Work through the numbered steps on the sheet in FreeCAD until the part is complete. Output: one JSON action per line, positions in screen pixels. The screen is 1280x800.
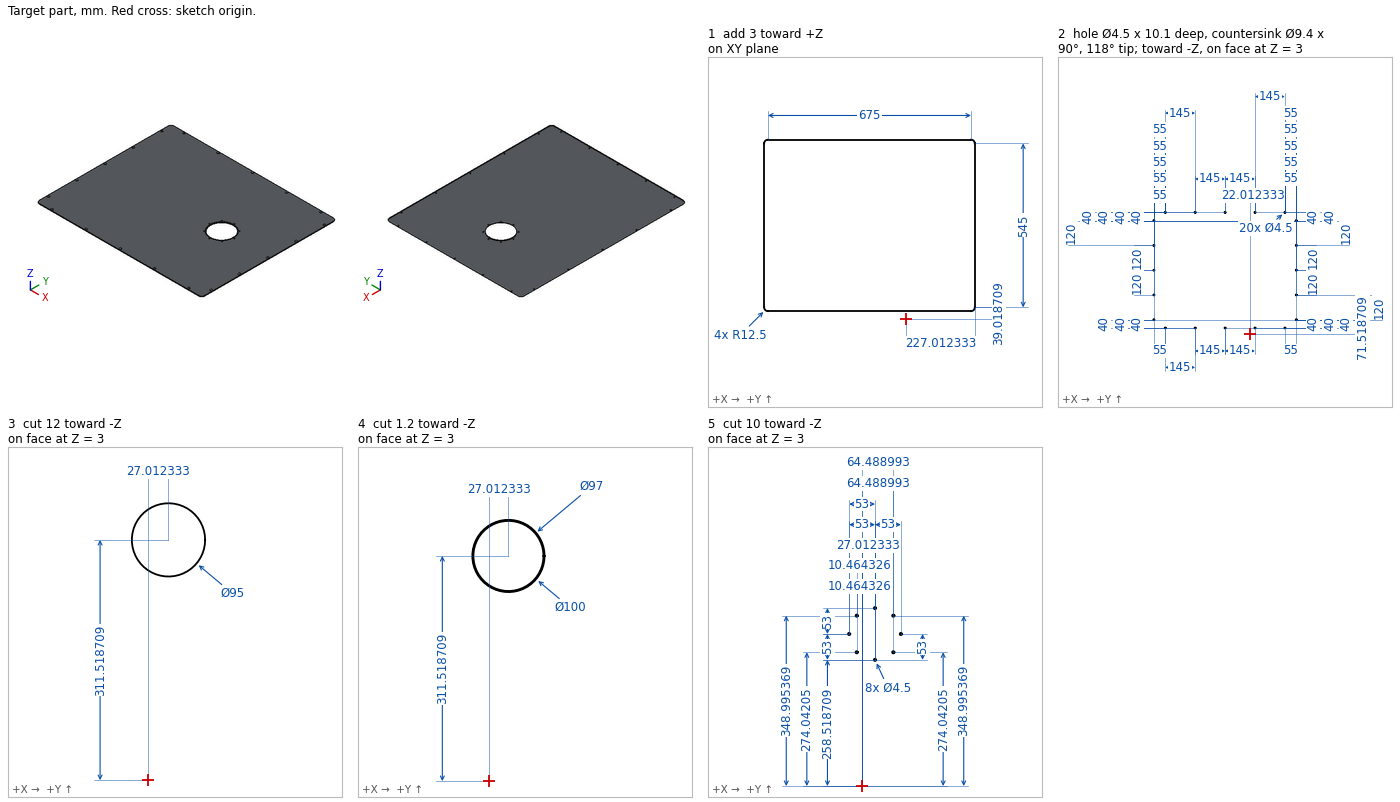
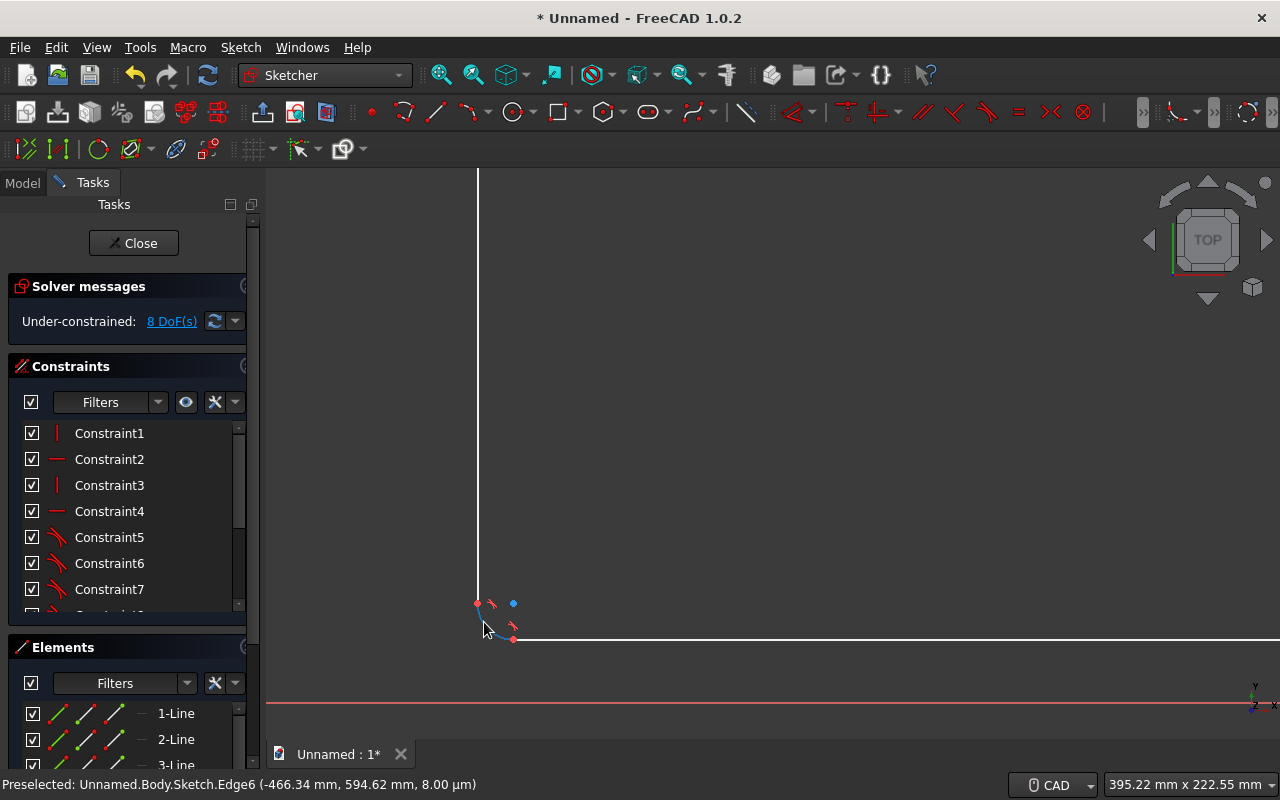
{"action": "left_click", "coordinate": [482, 620]}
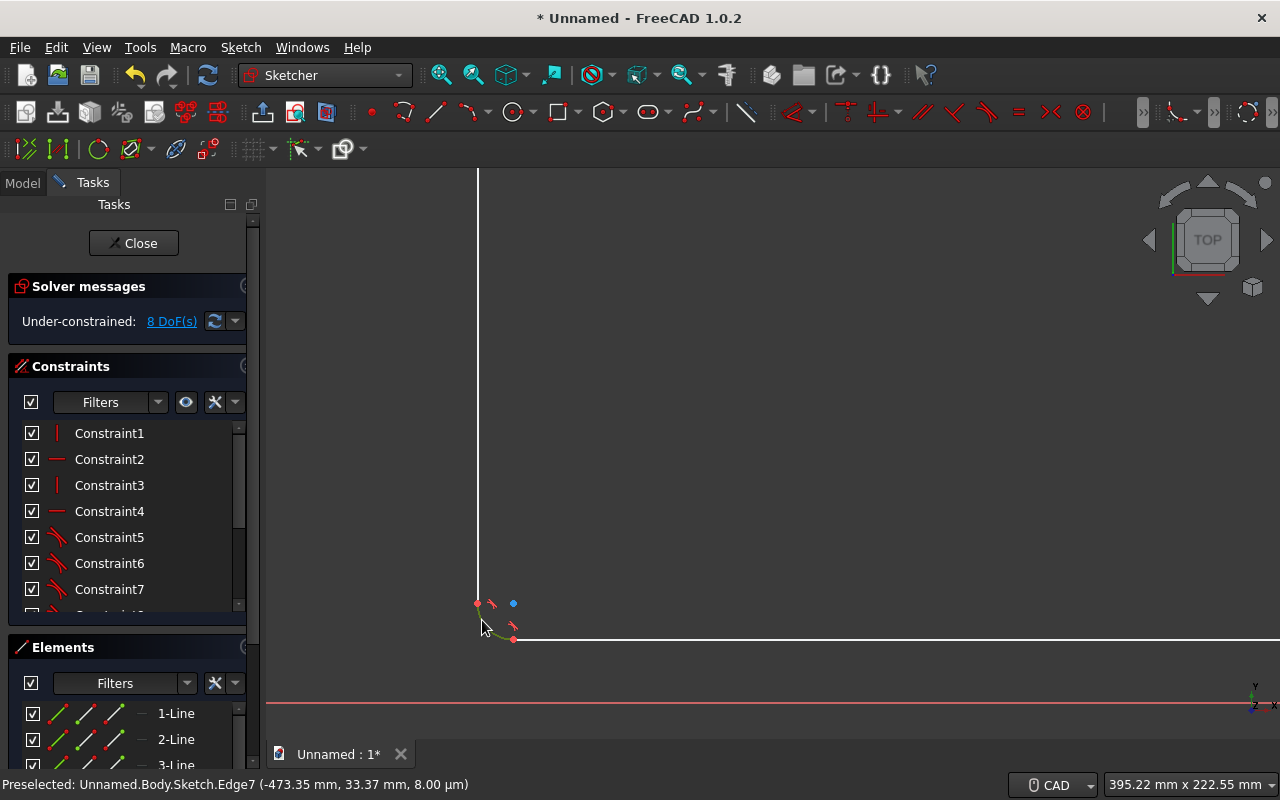
{"action": "scroll", "coordinate": [484, 622], "scroll_direction": "down", "scroll_amount": 7}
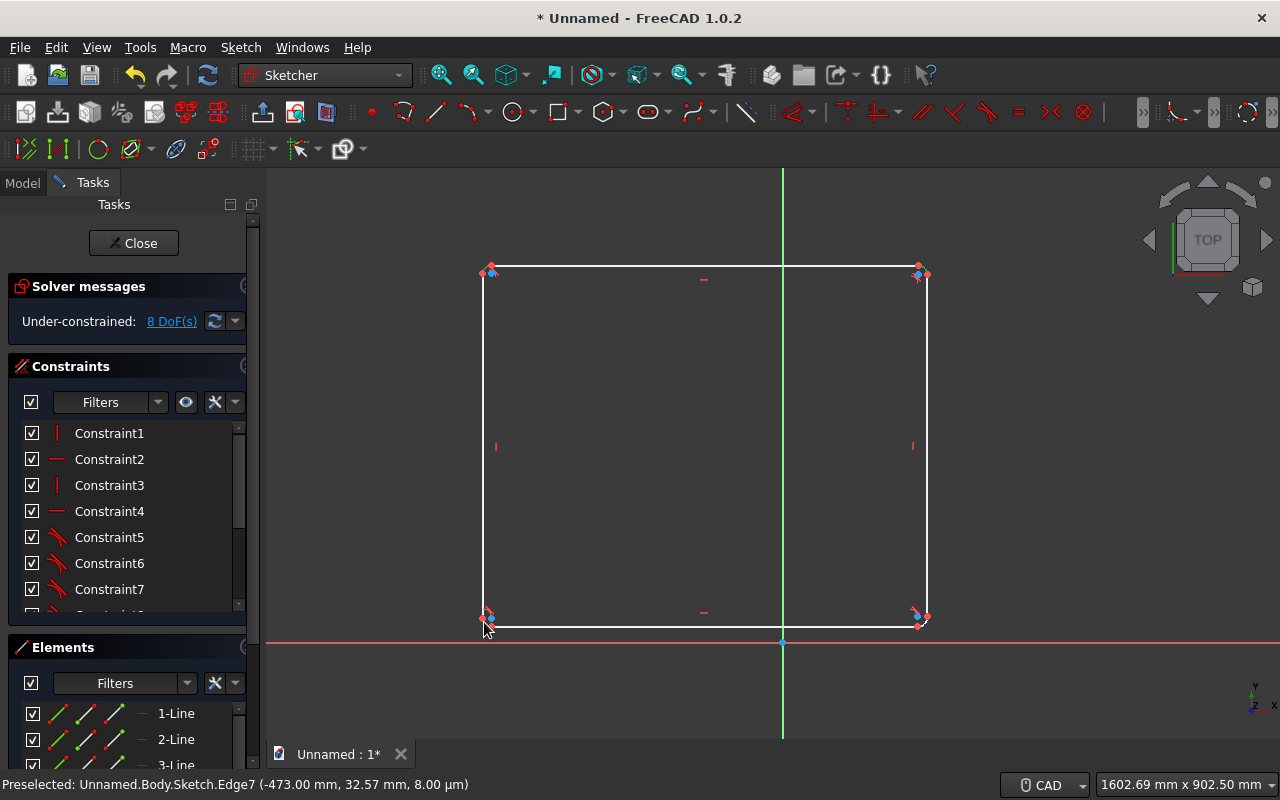
{"action": "scroll", "coordinate": [922, 626], "scroll_direction": "up", "scroll_amount": 6}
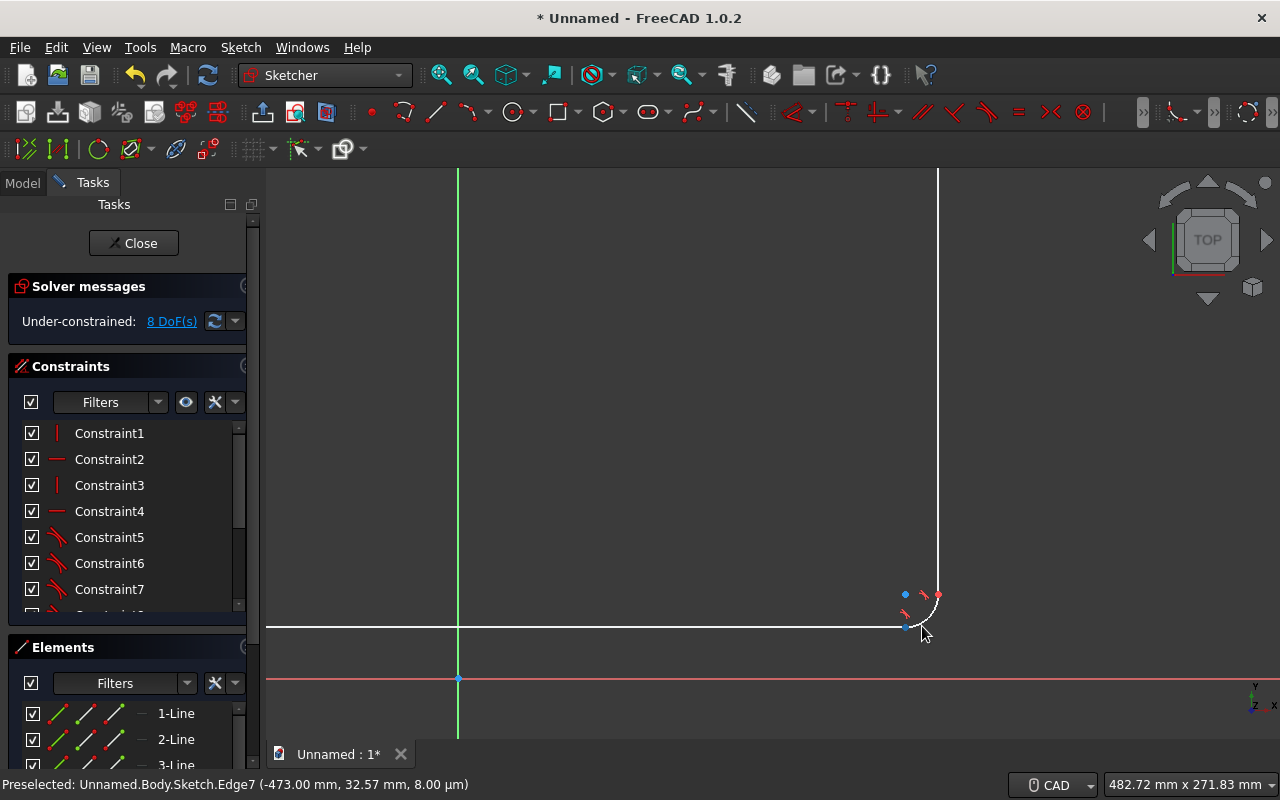
{"action": "left_click", "coordinate": [920, 624]}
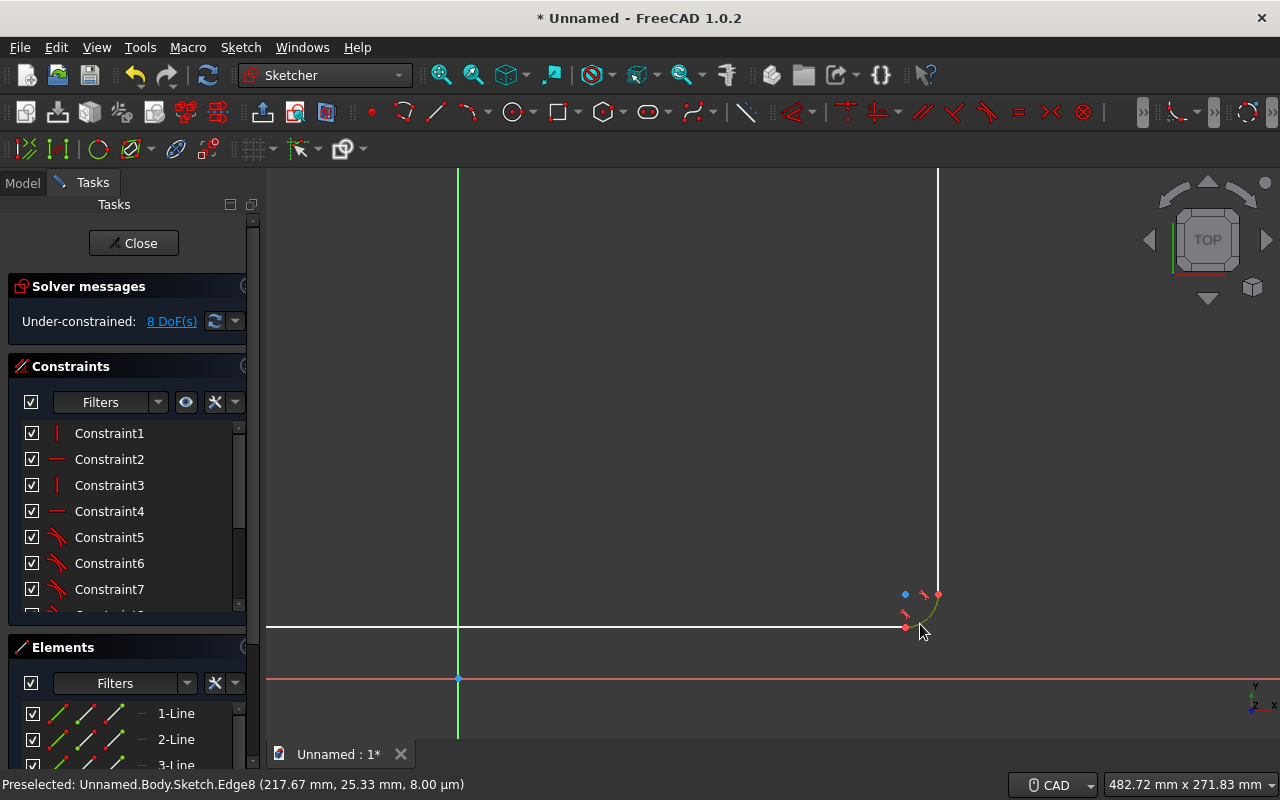
{"action": "left_click", "coordinate": [1020, 112]}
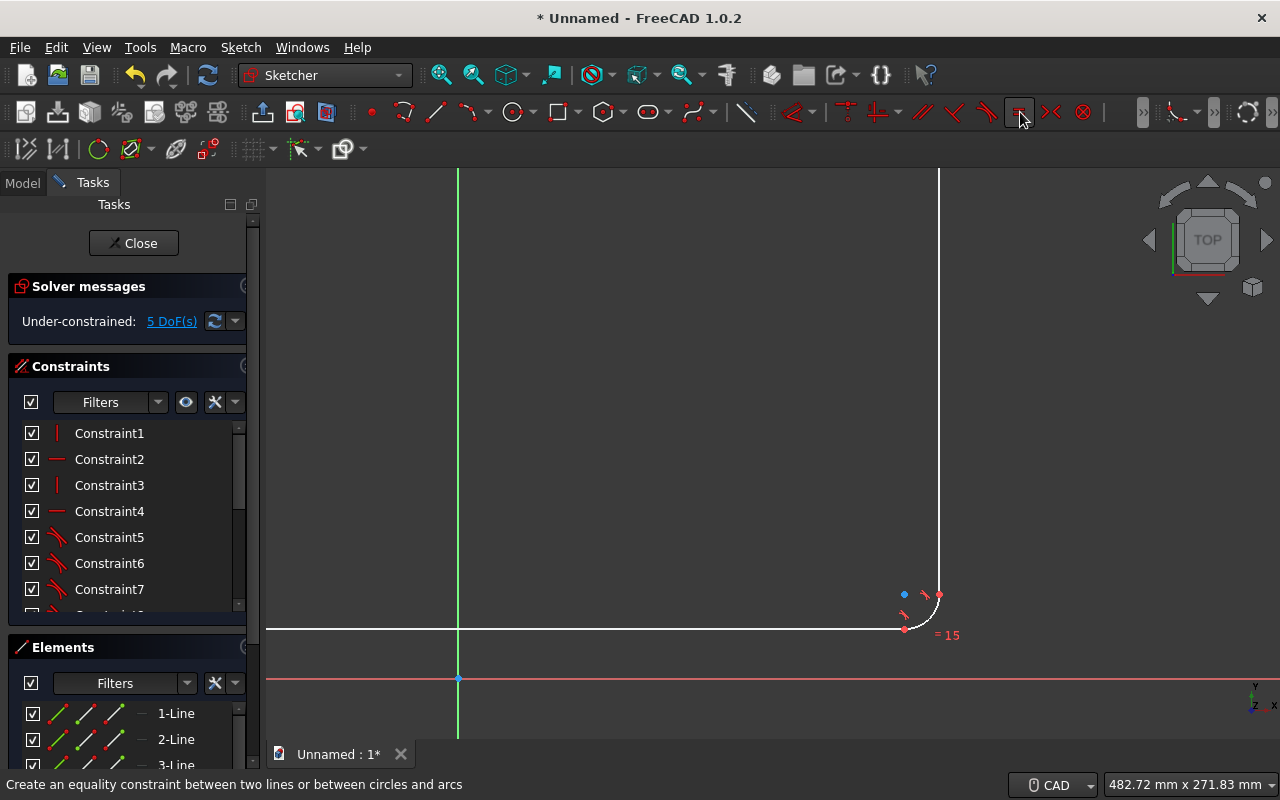
{"action": "scroll", "coordinate": [922, 626], "scroll_direction": "down", "scroll_amount": 6}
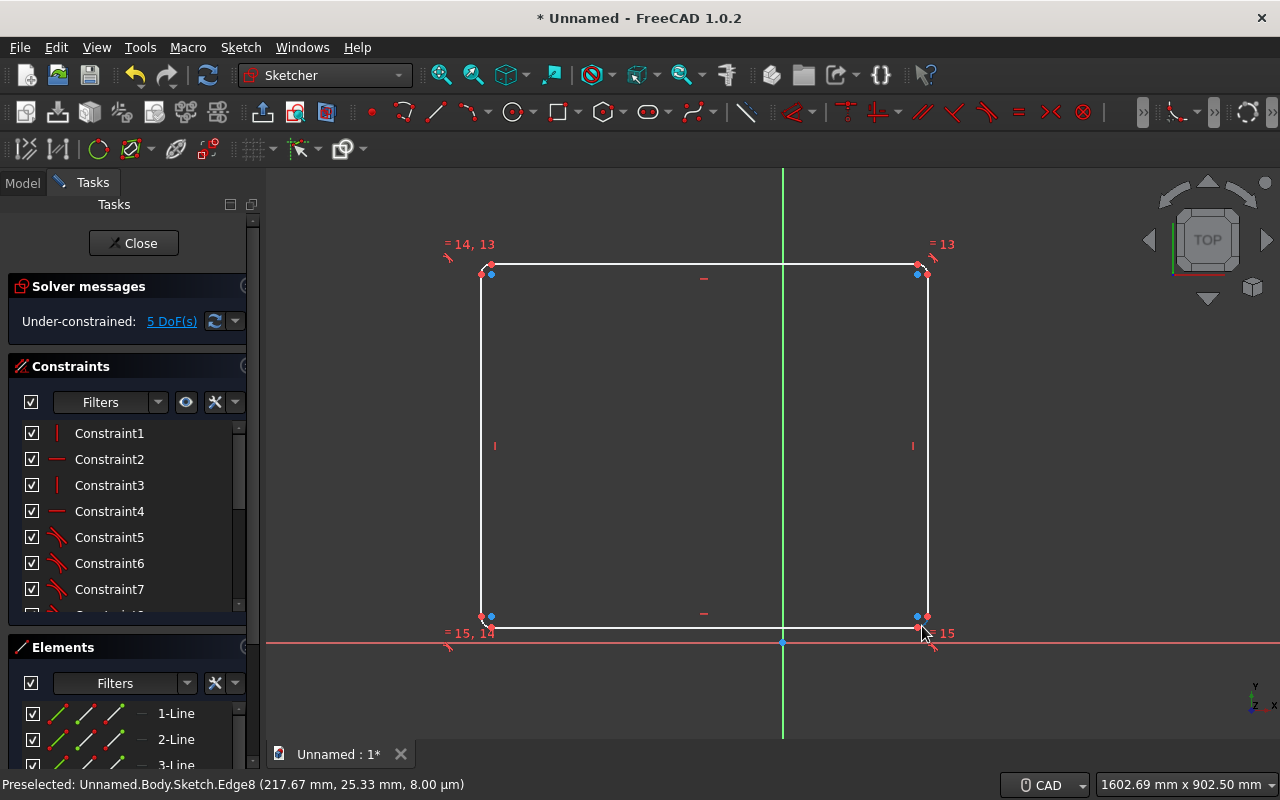
{"action": "scroll", "coordinate": [927, 270], "scroll_direction": "up", "scroll_amount": 9}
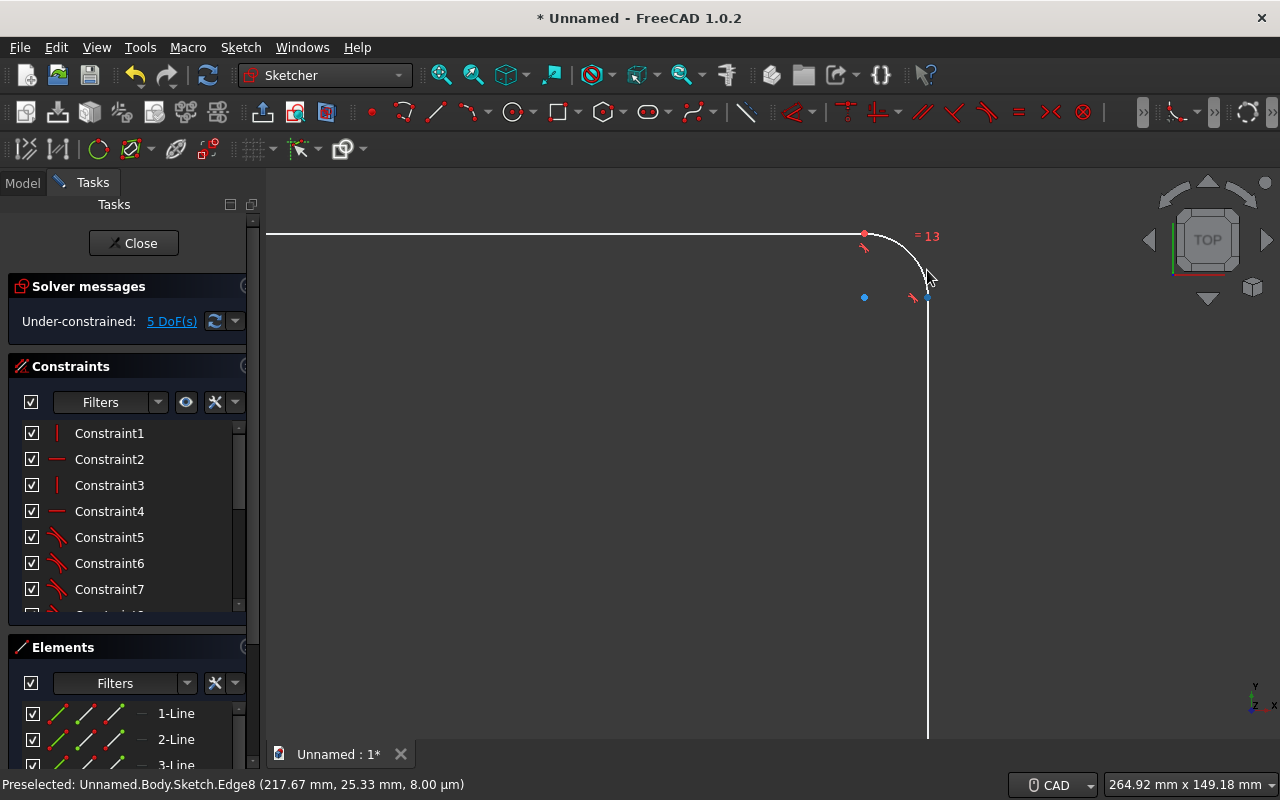
{"action": "left_click", "coordinate": [921, 269]}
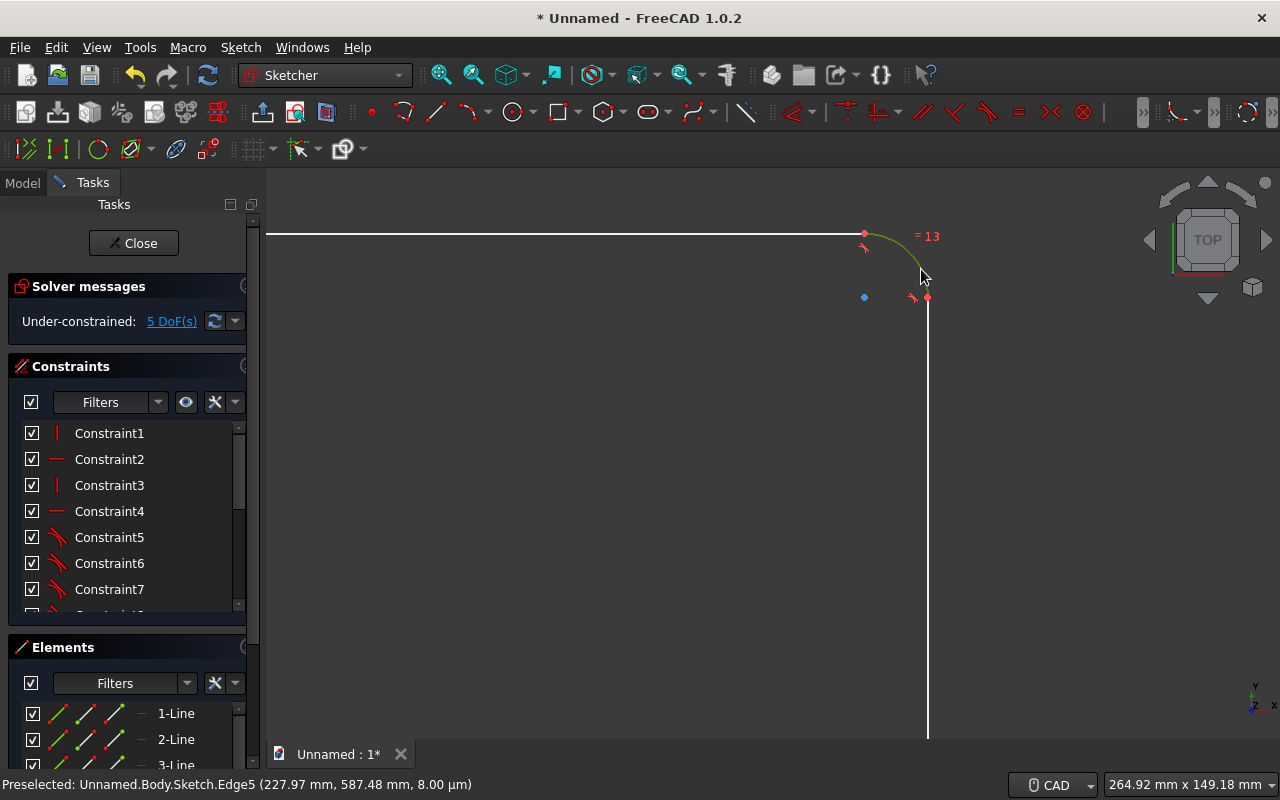
{"action": "left_click", "coordinate": [814, 112]}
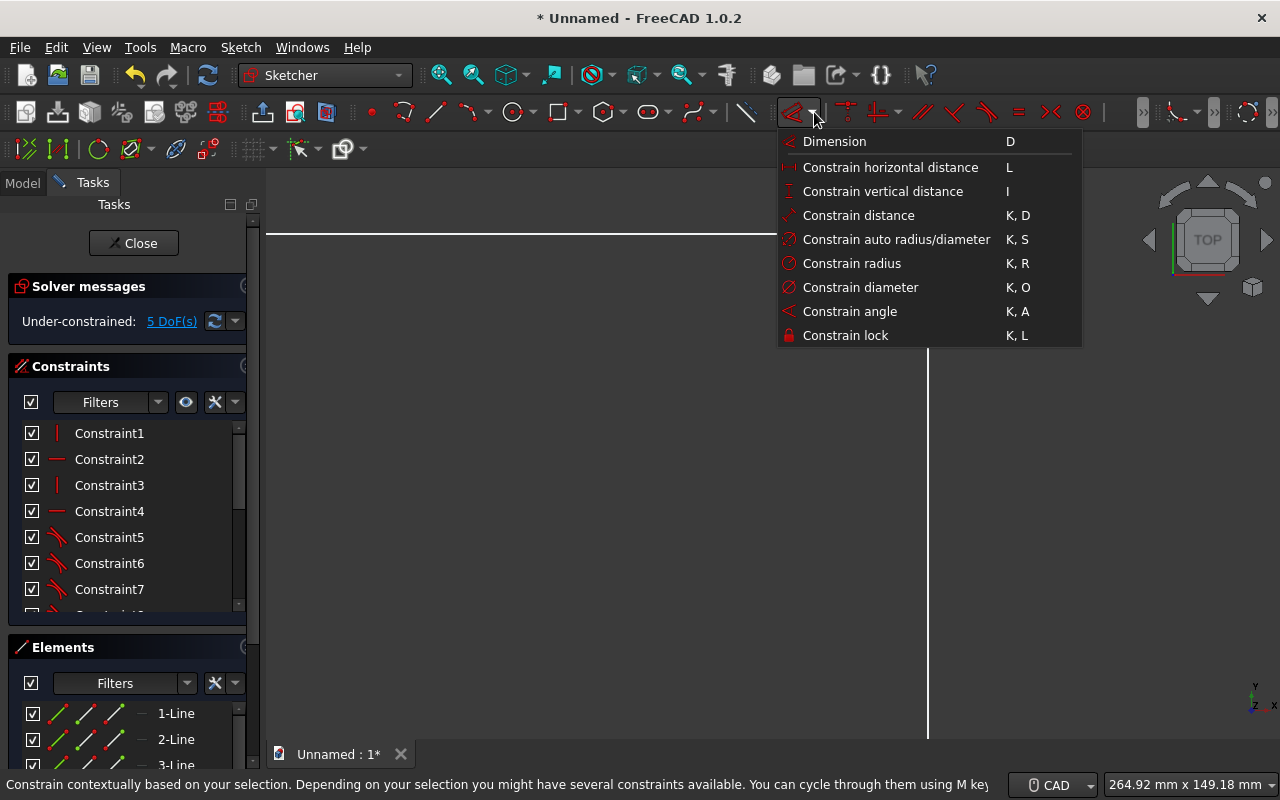
{"action": "left_click", "coordinate": [930, 263]}